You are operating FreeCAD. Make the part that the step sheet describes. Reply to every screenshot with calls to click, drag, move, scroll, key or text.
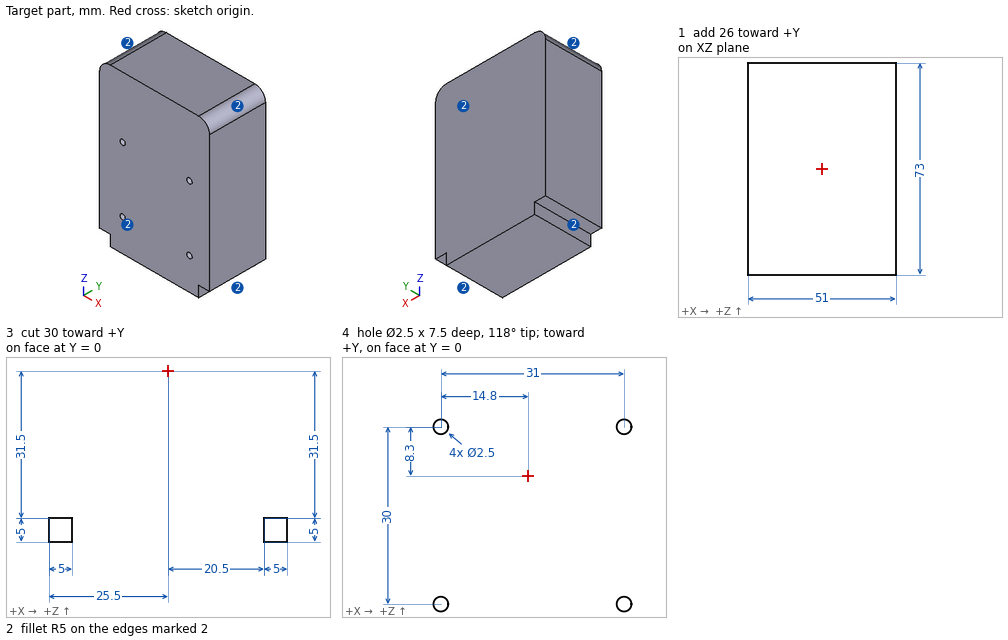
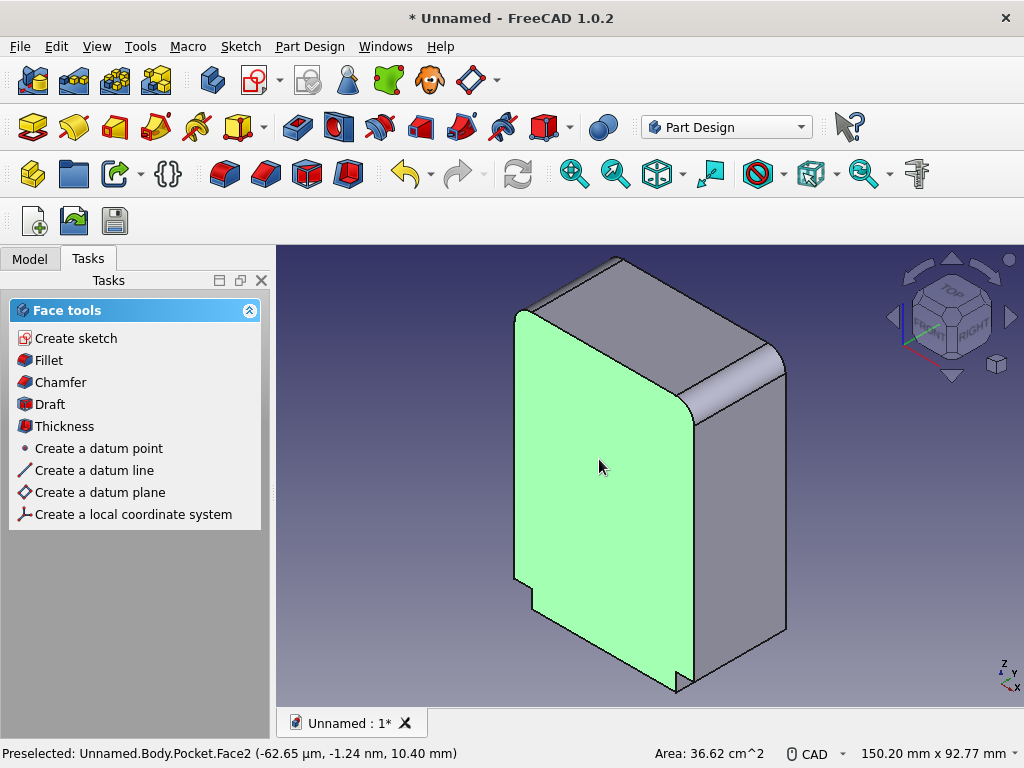
click(254, 80)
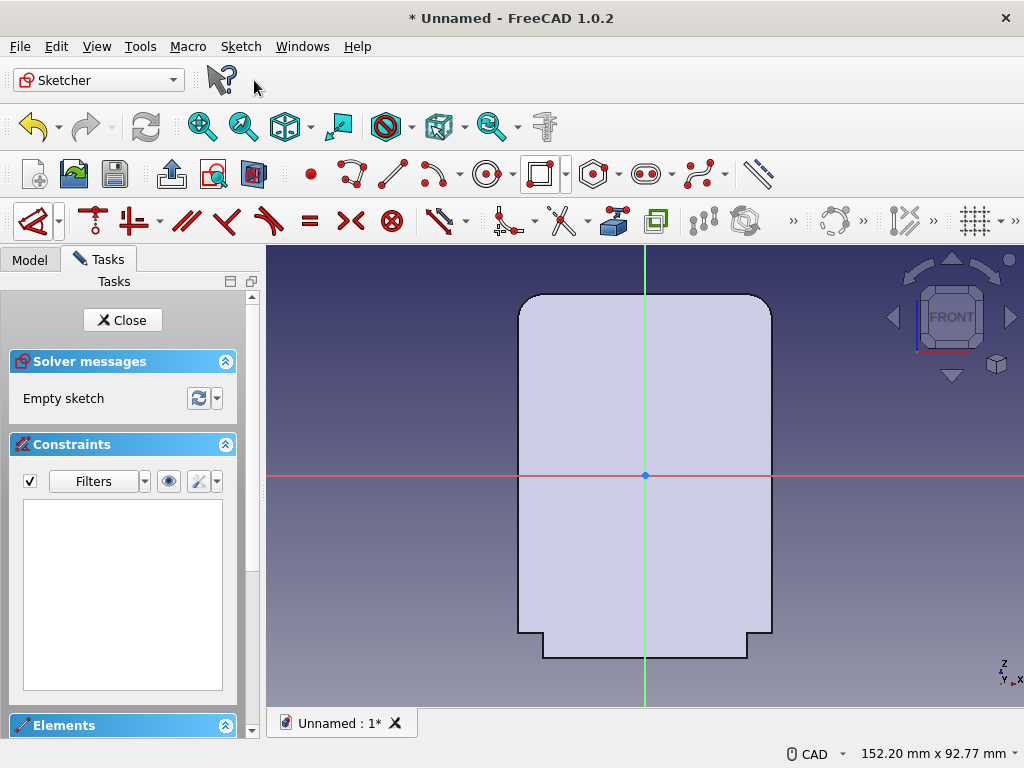
scroll(736, 550, up, 3)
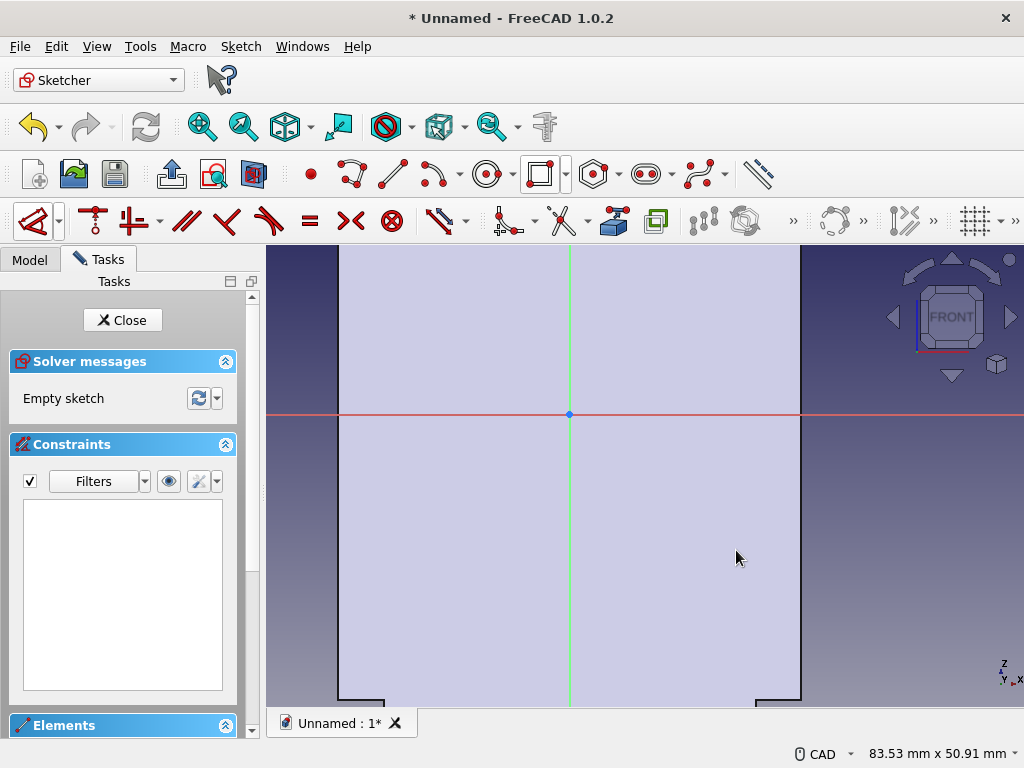
click(486, 174)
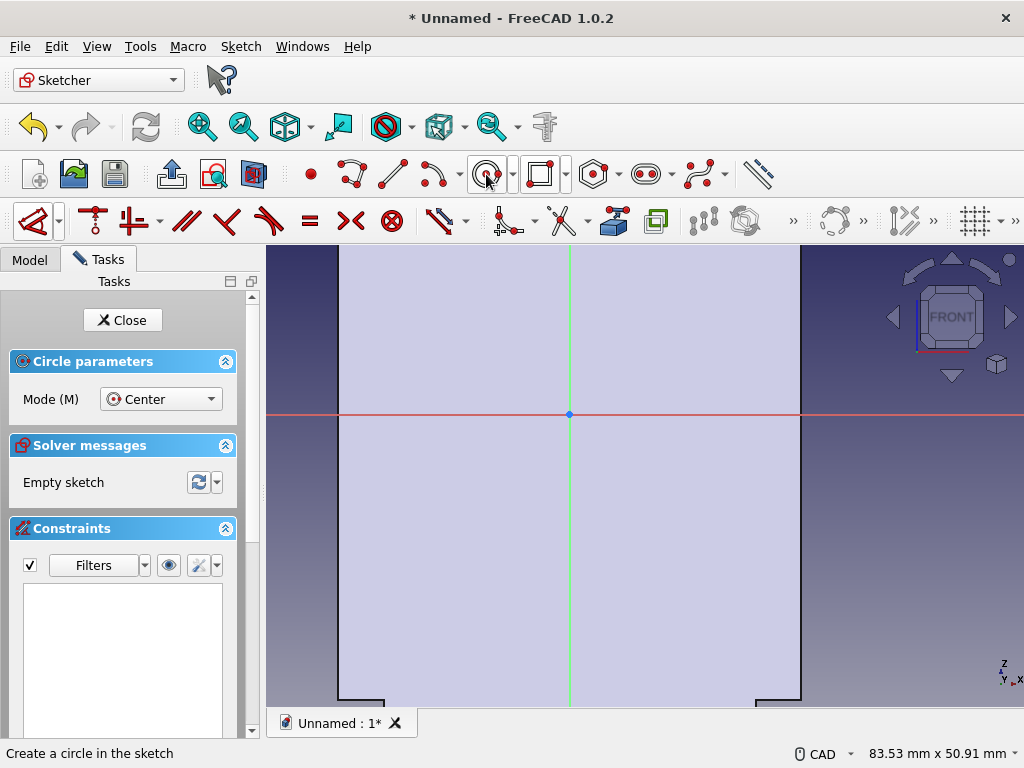
scroll(435, 339, up, 4)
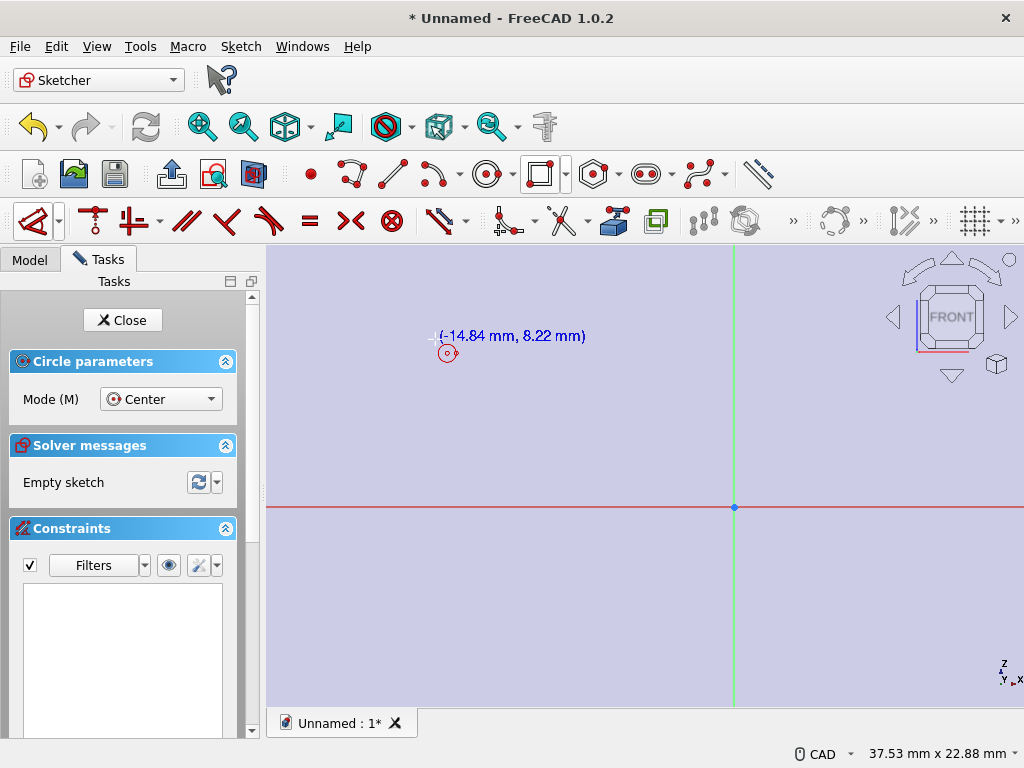
click(436, 339)
click(453, 322)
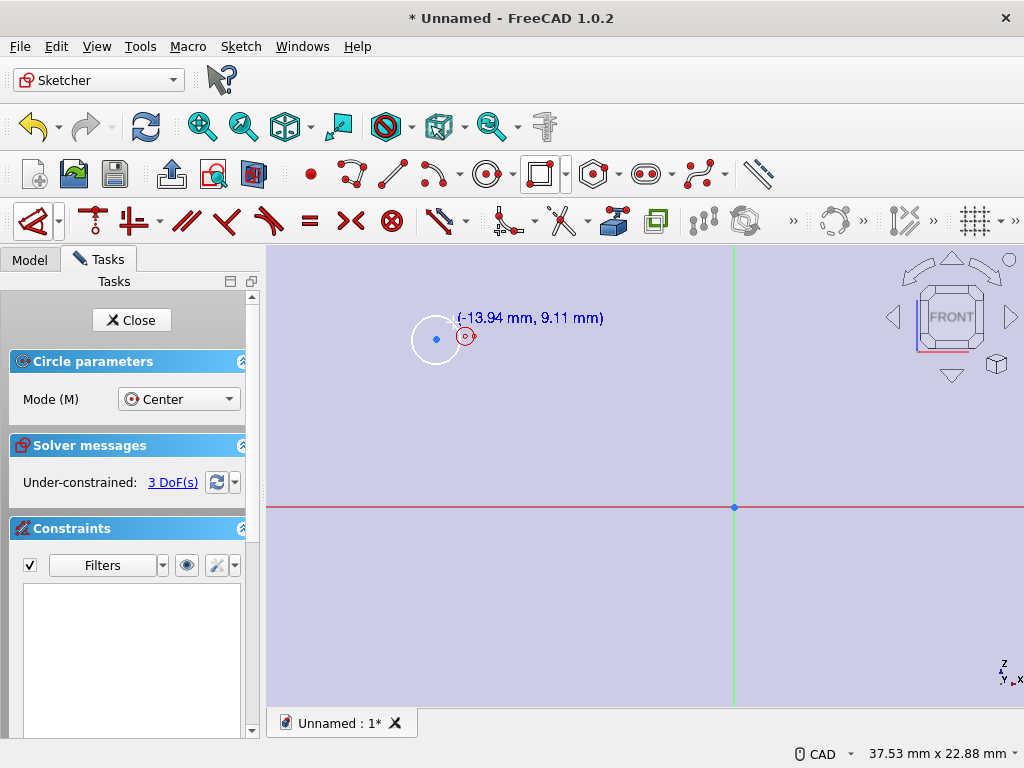
scroll(436, 340, down, 4)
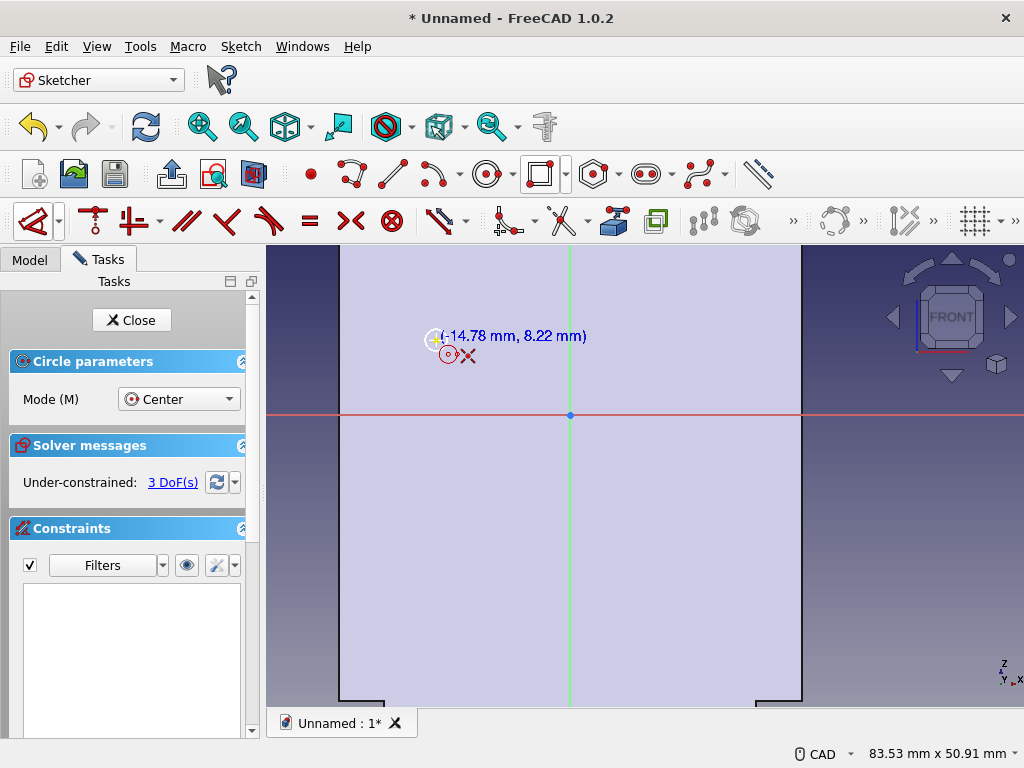
scroll(717, 340, up, 4)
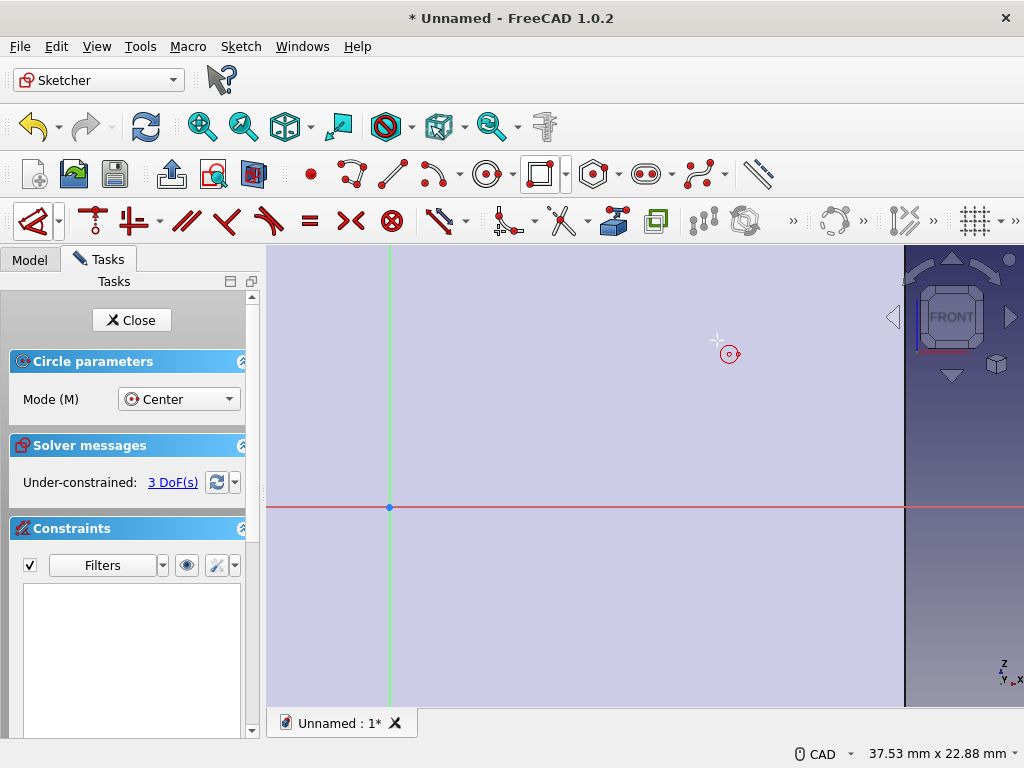
click(717, 339)
click(735, 322)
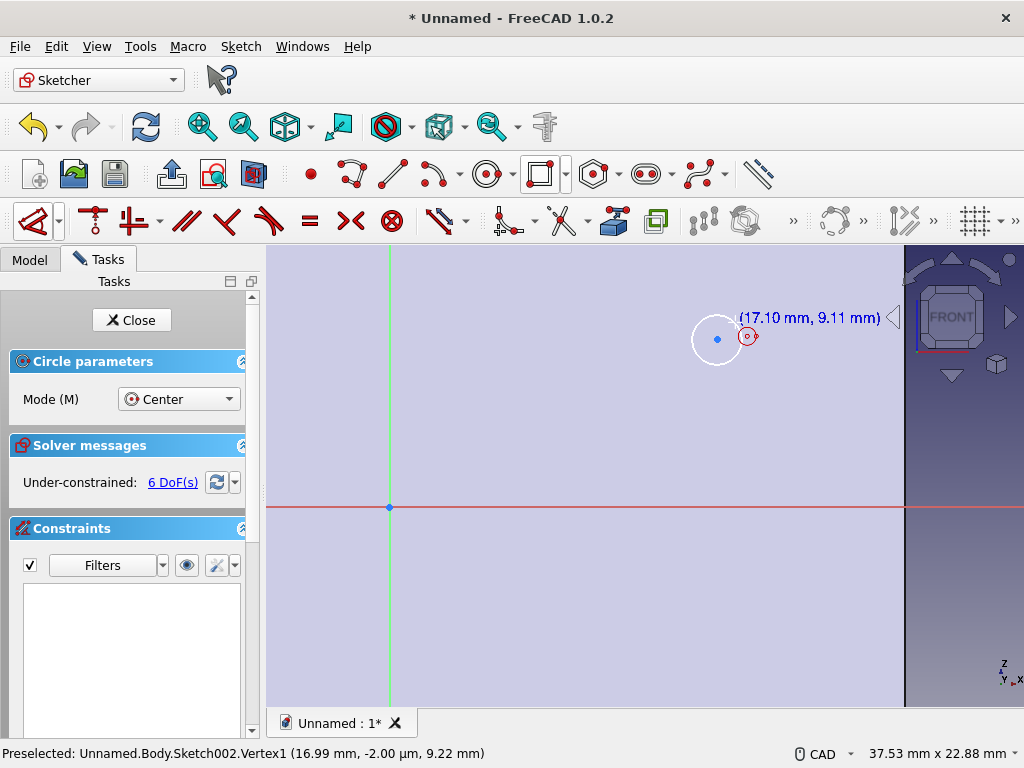
scroll(717, 340, down, 4)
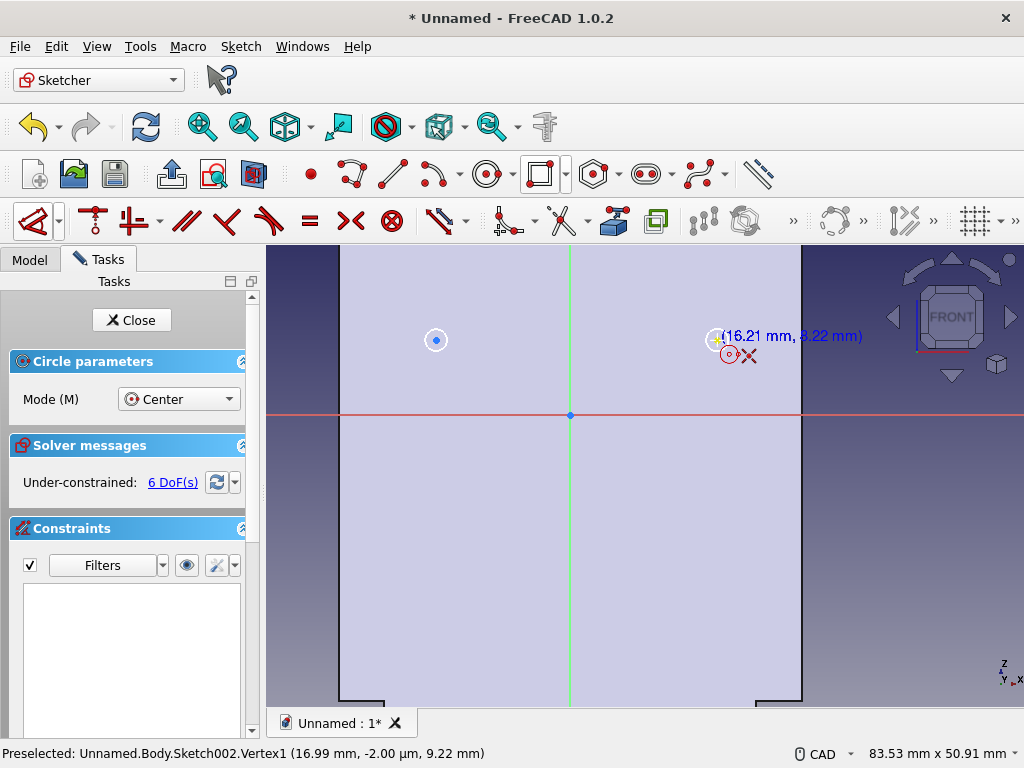
scroll(436, 612, up, 4)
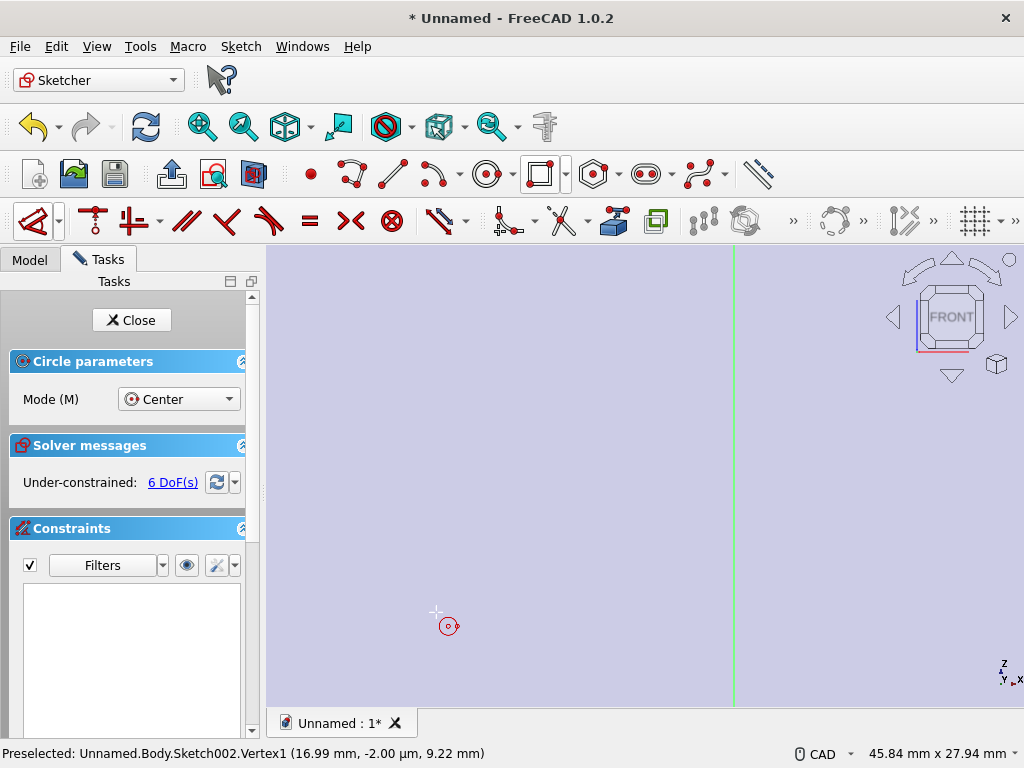
click(436, 611)
click(453, 593)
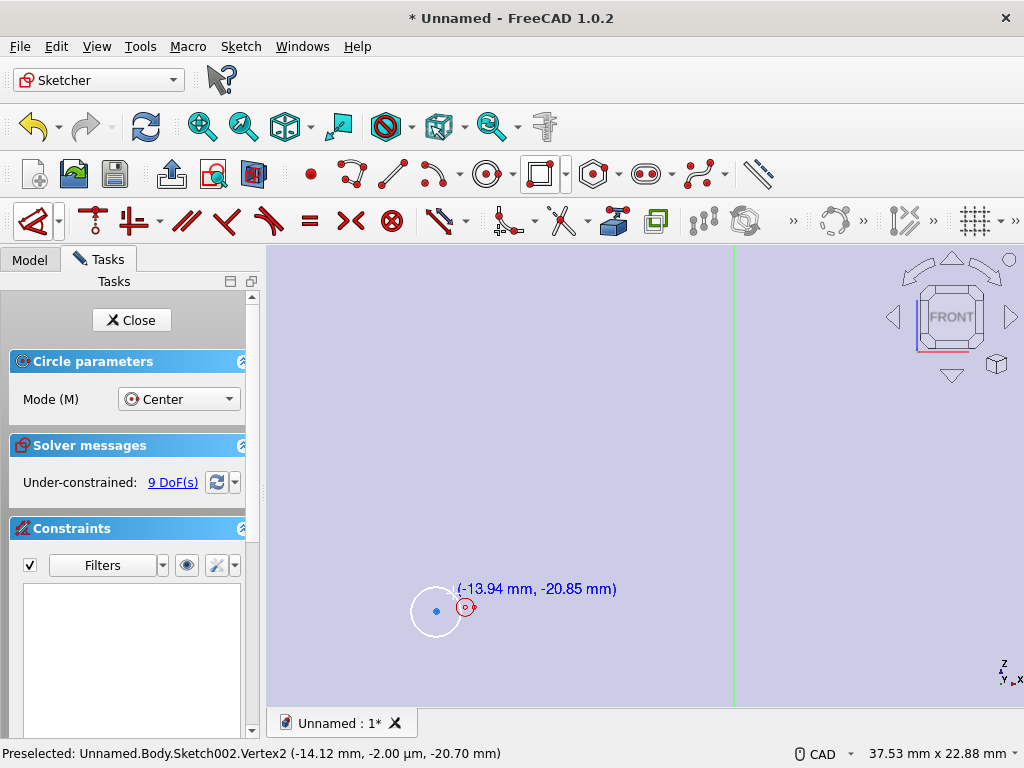
scroll(436, 613, down, 4)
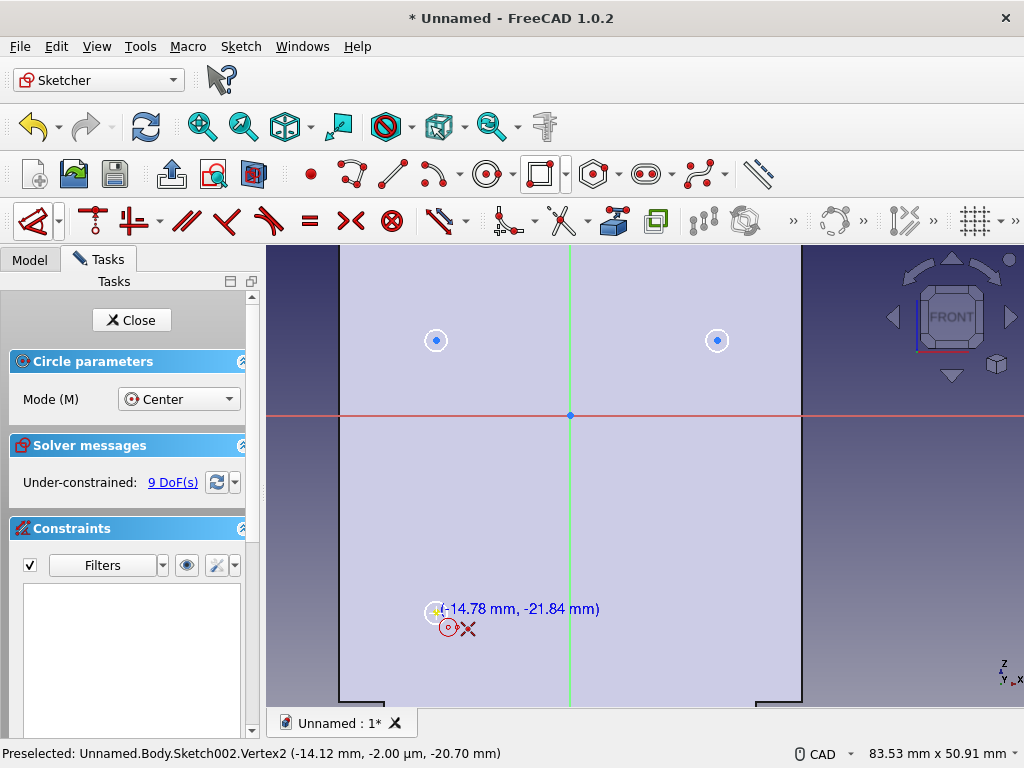
scroll(717, 613, up, 4)